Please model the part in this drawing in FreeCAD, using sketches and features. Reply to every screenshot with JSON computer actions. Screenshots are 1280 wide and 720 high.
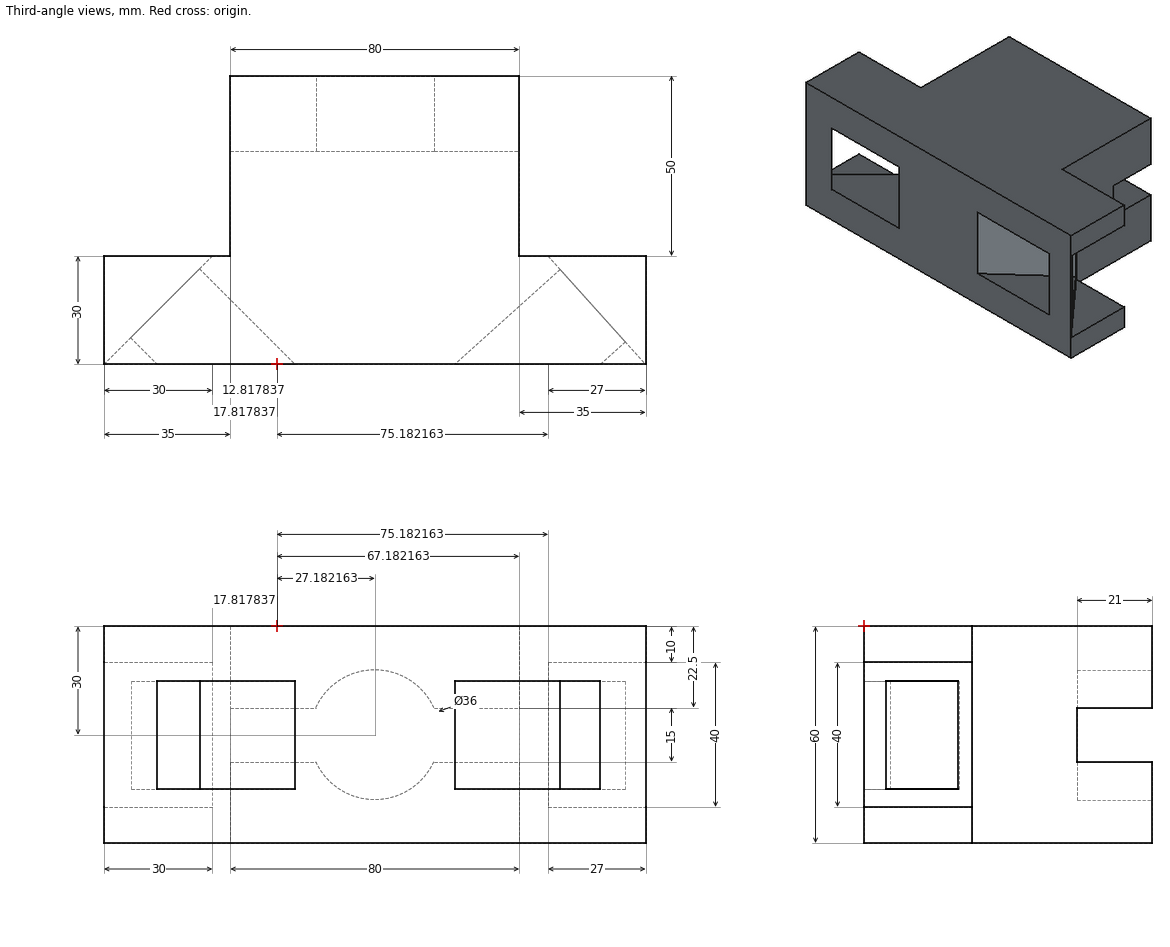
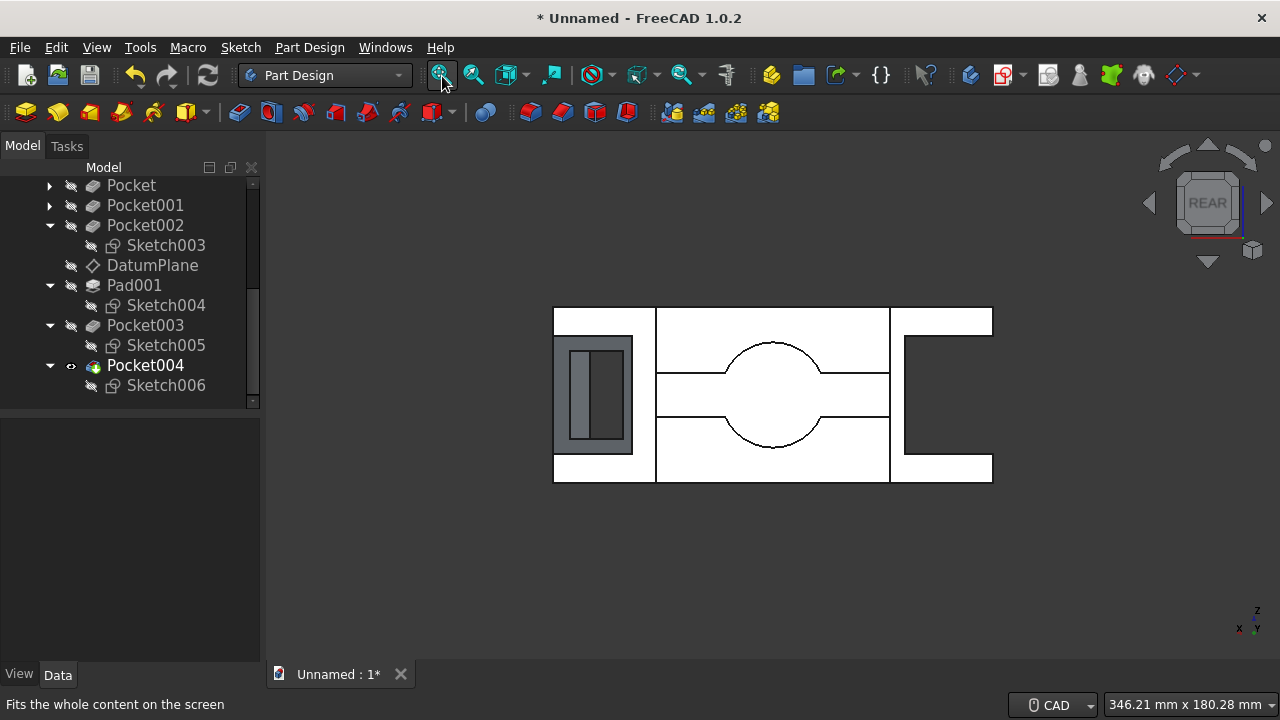
{"action": "scroll", "coordinate": [140, 281], "scroll_direction": "down", "scroll_amount": 3}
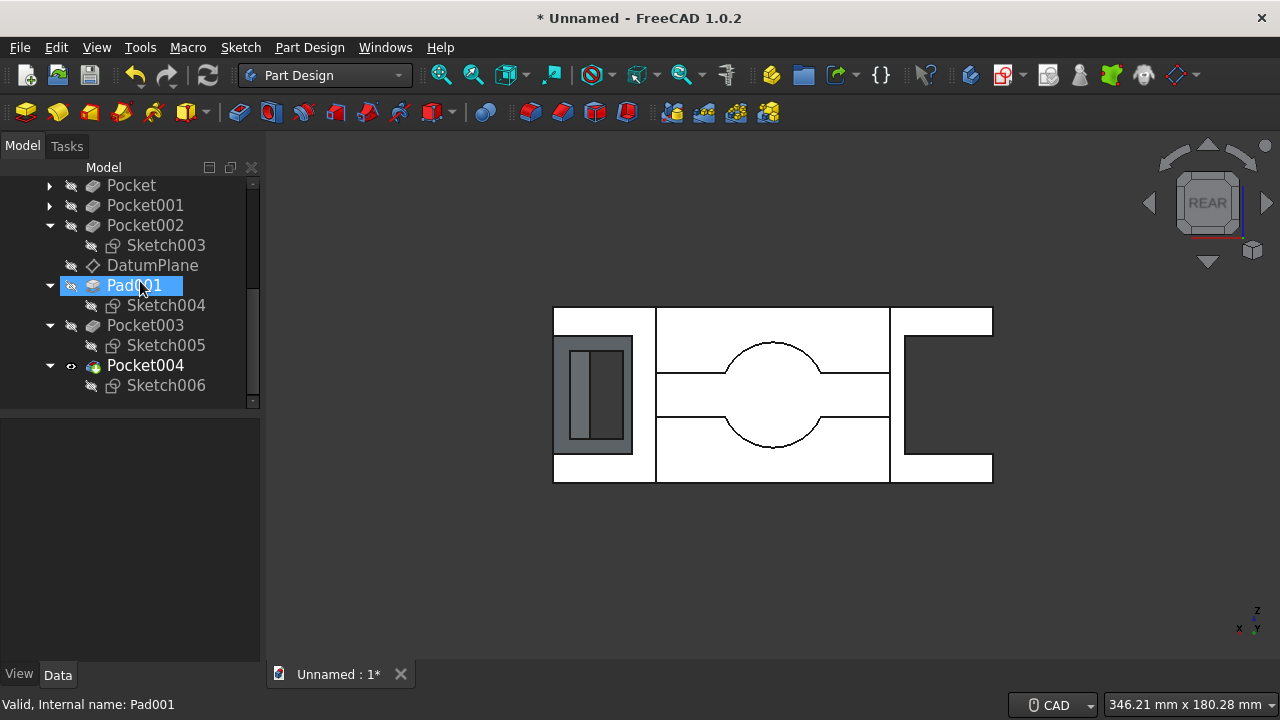
{"action": "scroll", "coordinate": [140, 281], "scroll_direction": "up", "scroll_amount": 15}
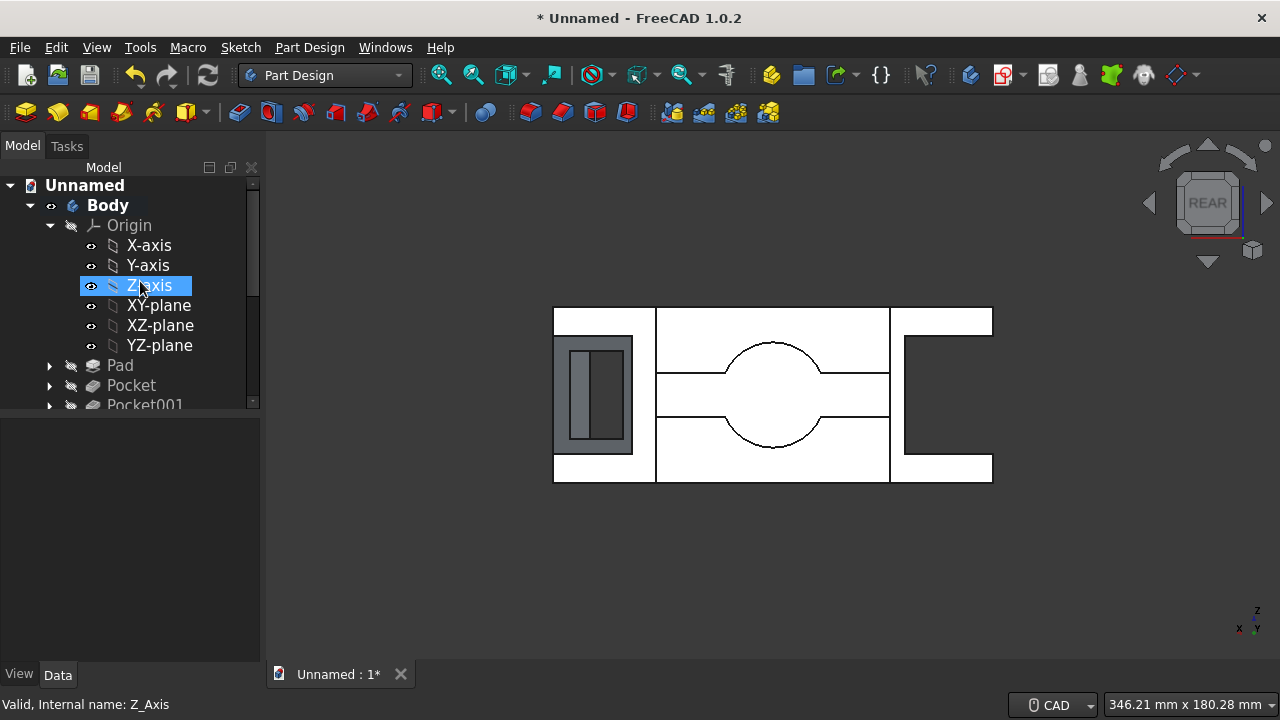
{"action": "left_click", "coordinate": [136, 306]}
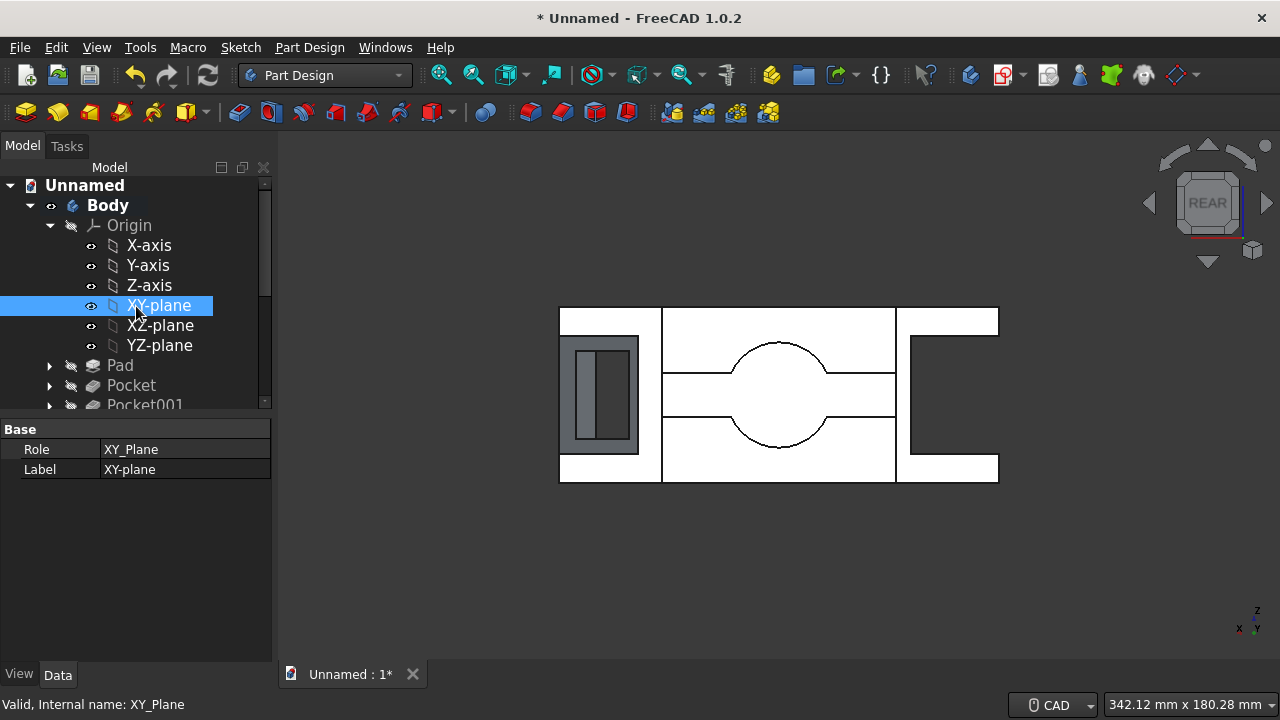
{"action": "left_click", "coordinate": [1176, 76]}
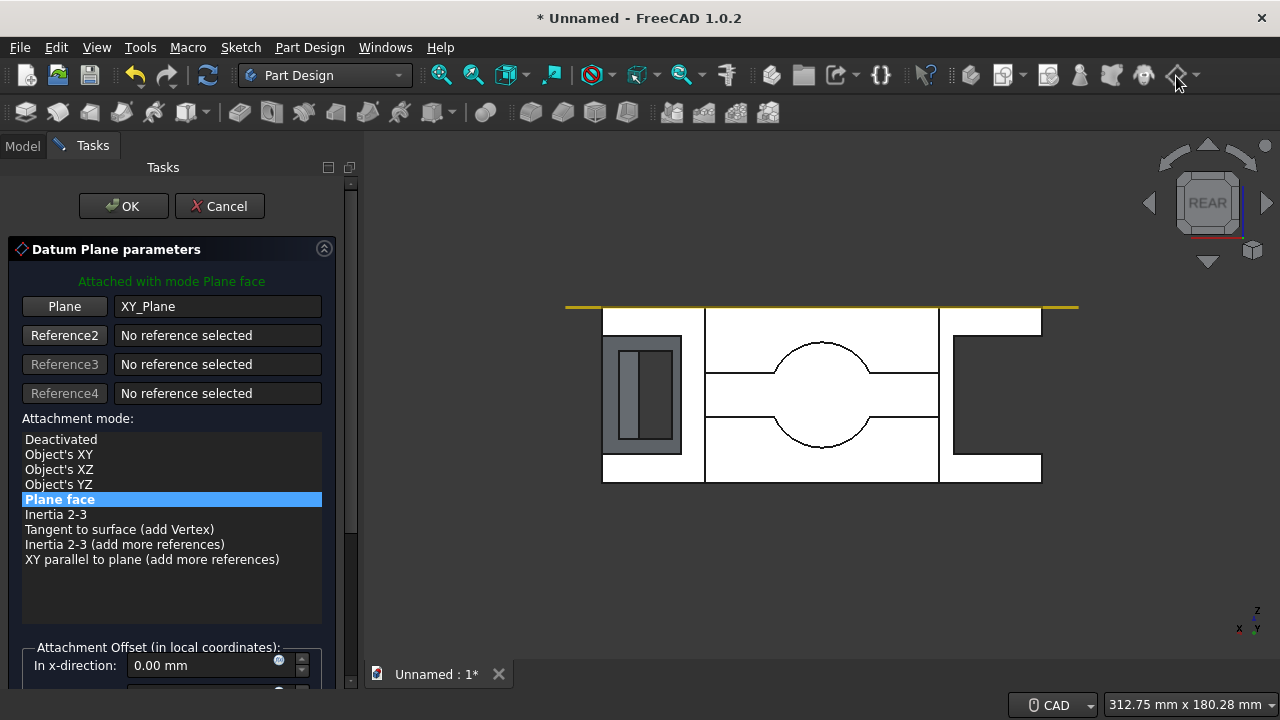
{"action": "scroll", "coordinate": [351, 432], "scroll_direction": "down", "scroll_amount": 2}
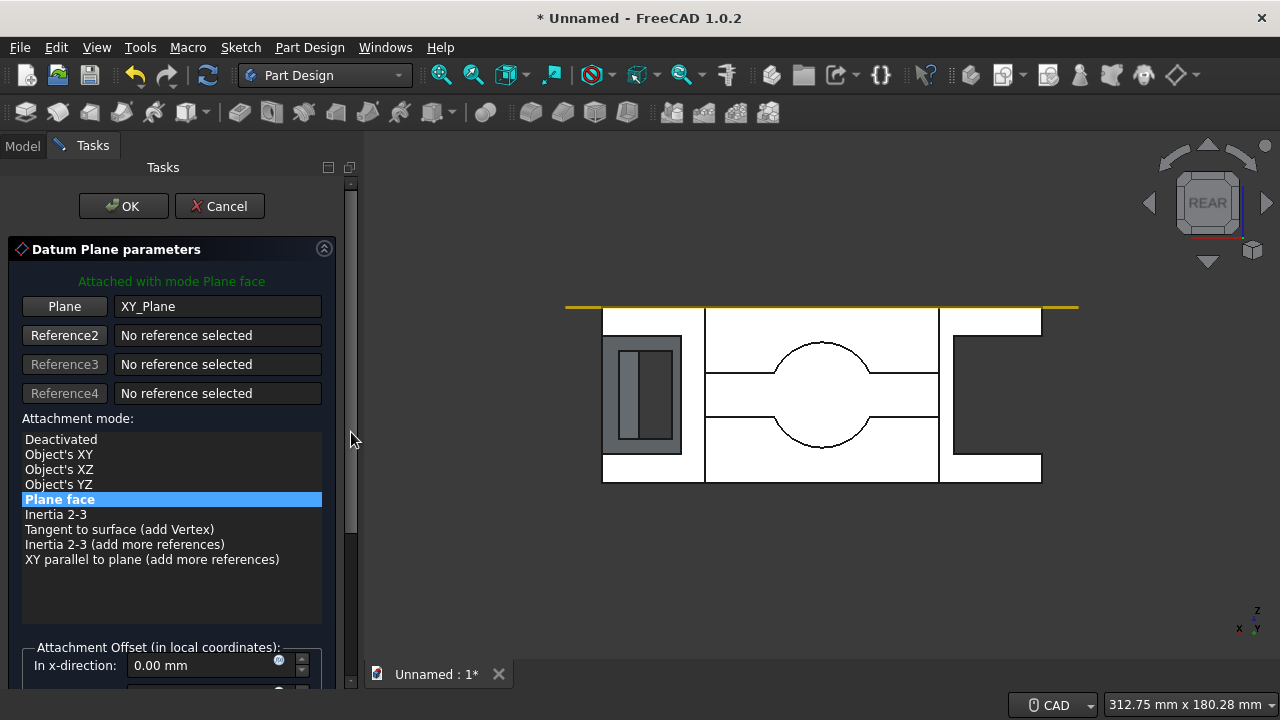
{"action": "triple_click", "coordinate": [210, 609]}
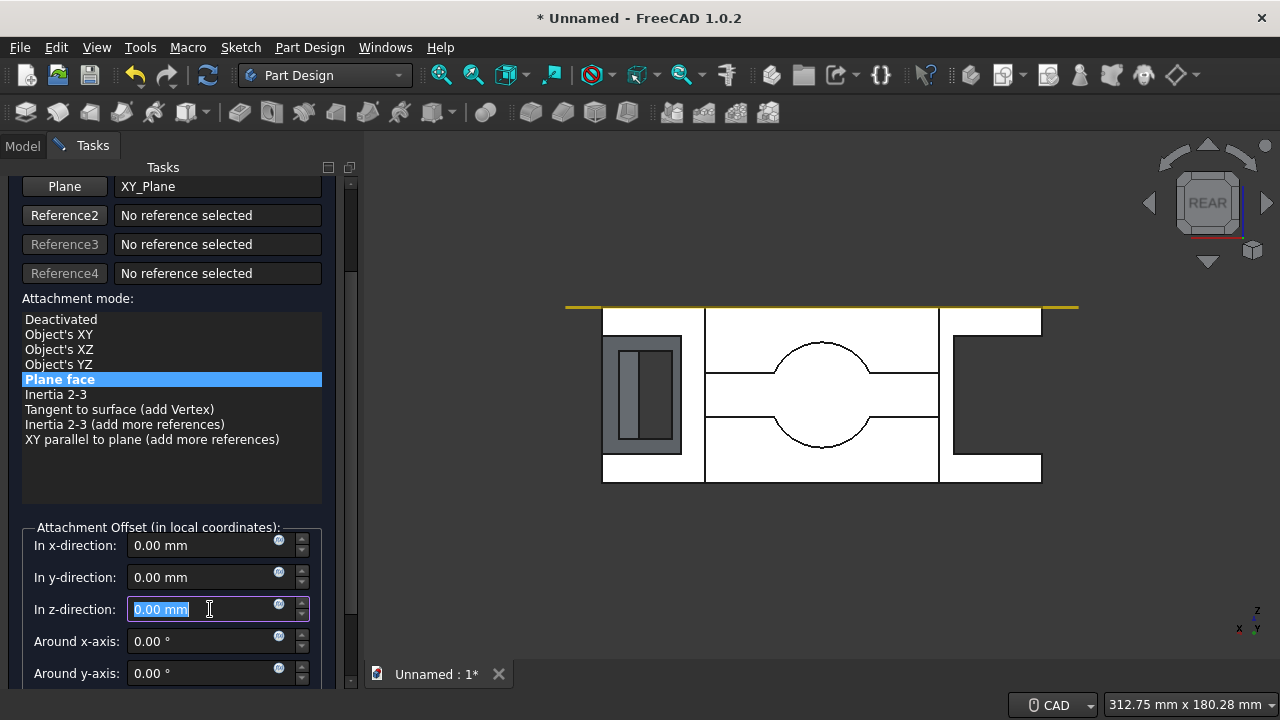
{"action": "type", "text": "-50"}
{"action": "key", "text": "Tab"}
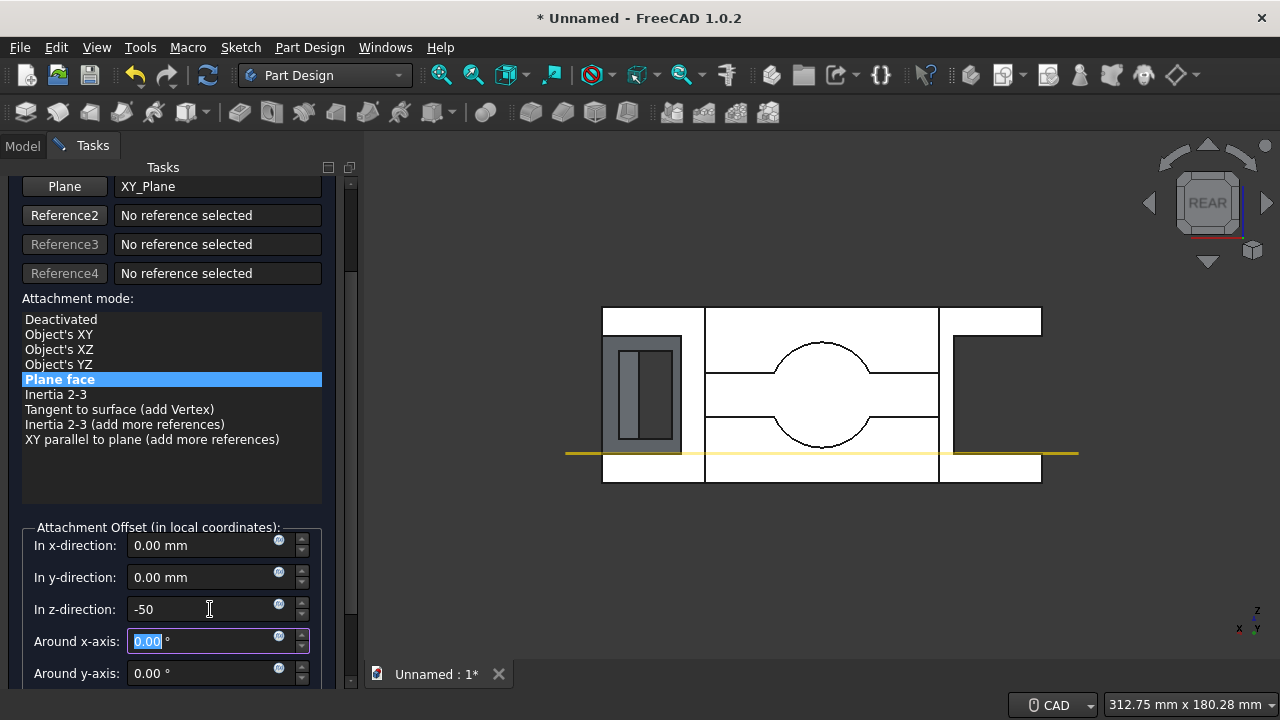
{"action": "scroll", "coordinate": [351, 432], "scroll_direction": "up", "scroll_amount": 3}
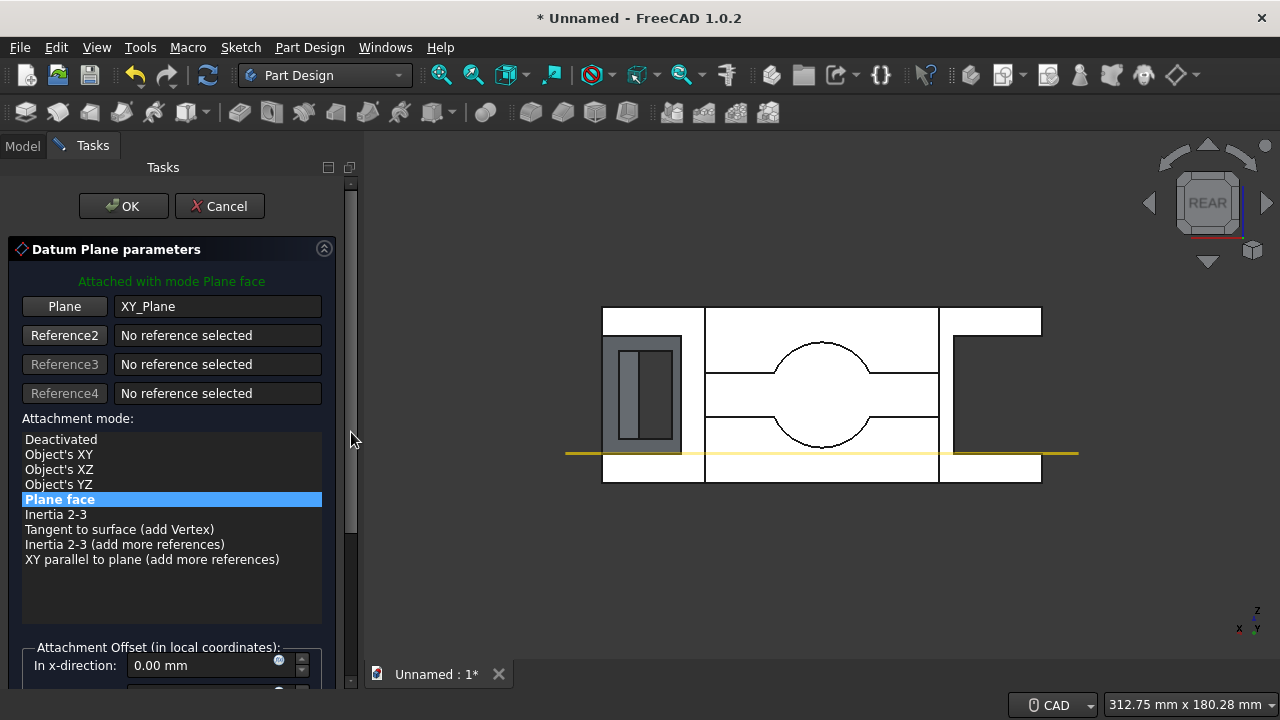
{"action": "left_click", "coordinate": [124, 206]}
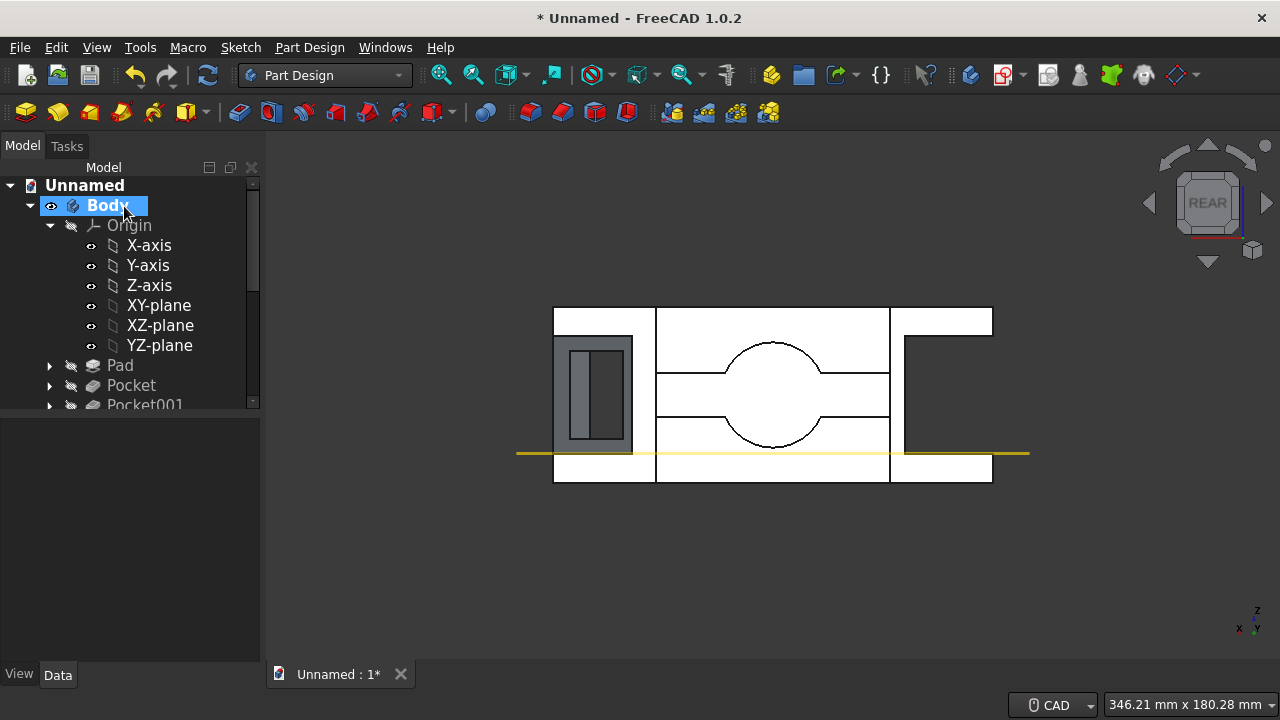
{"action": "scroll", "coordinate": [100, 301], "scroll_direction": "down", "scroll_amount": 3}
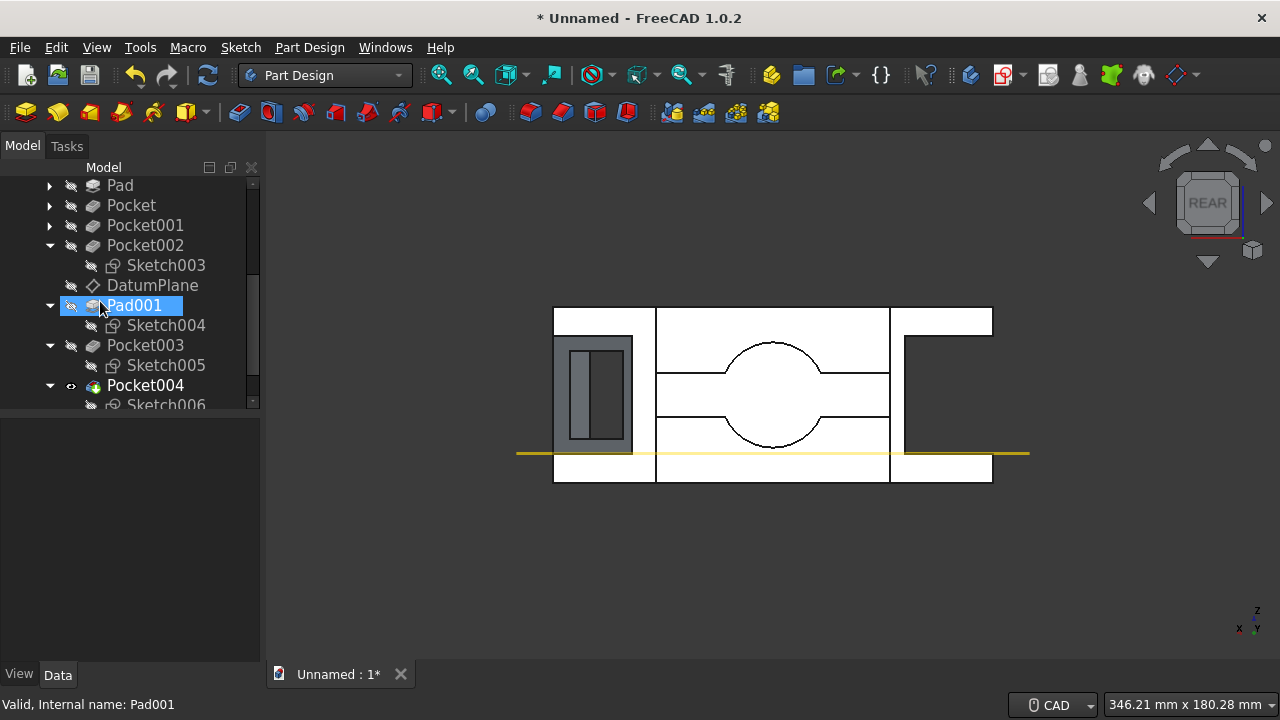
{"action": "scroll", "coordinate": [140, 301], "scroll_direction": "up", "scroll_amount": 15}